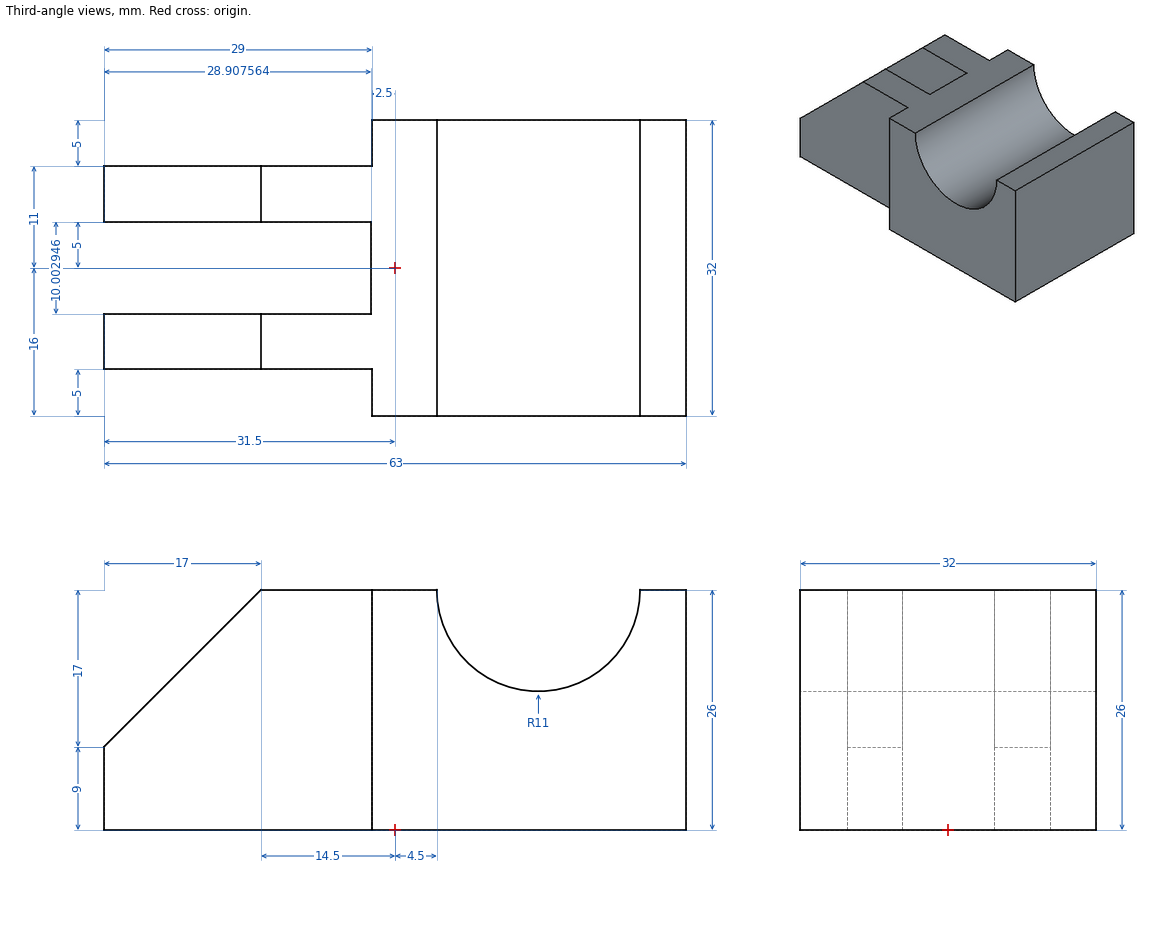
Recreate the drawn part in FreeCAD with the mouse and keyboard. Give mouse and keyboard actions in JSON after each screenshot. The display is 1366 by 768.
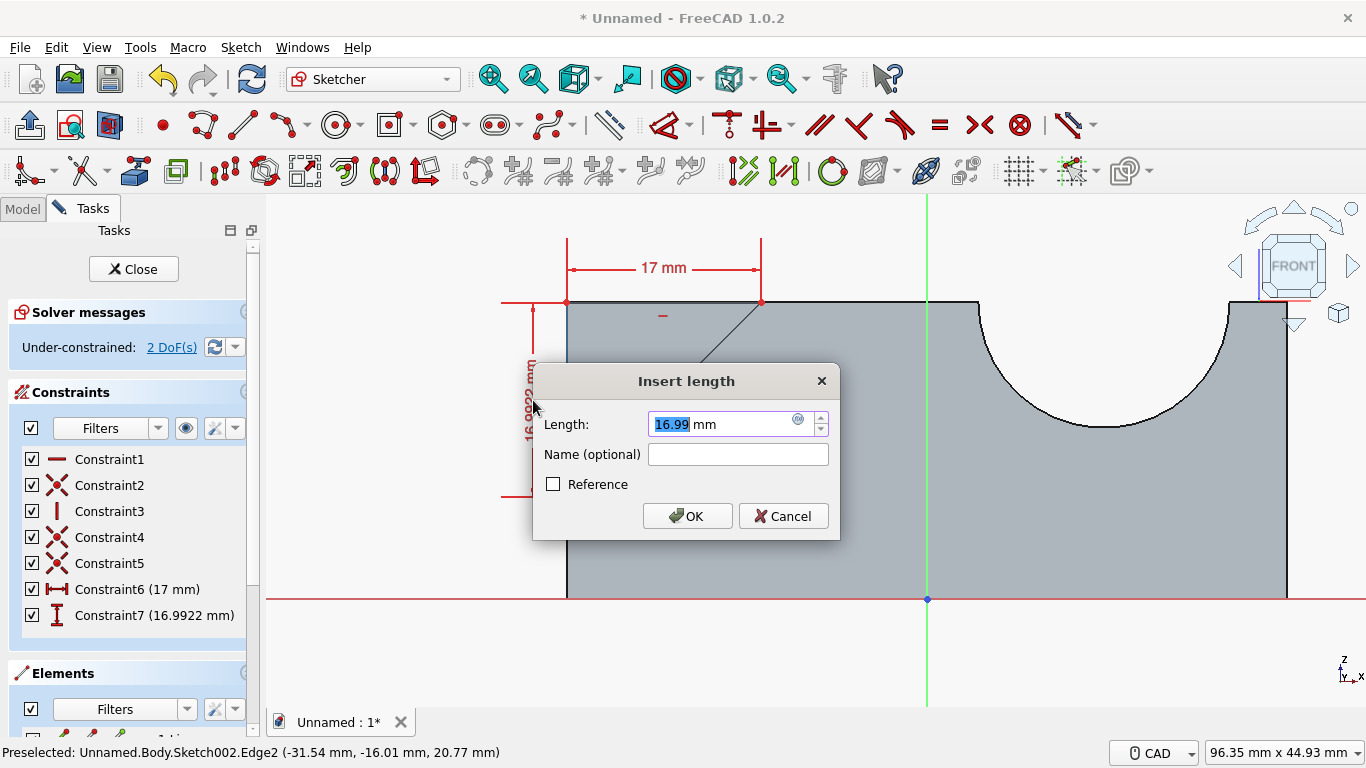
{"action": "type", "text": "17"}
{"action": "key", "text": "Return"}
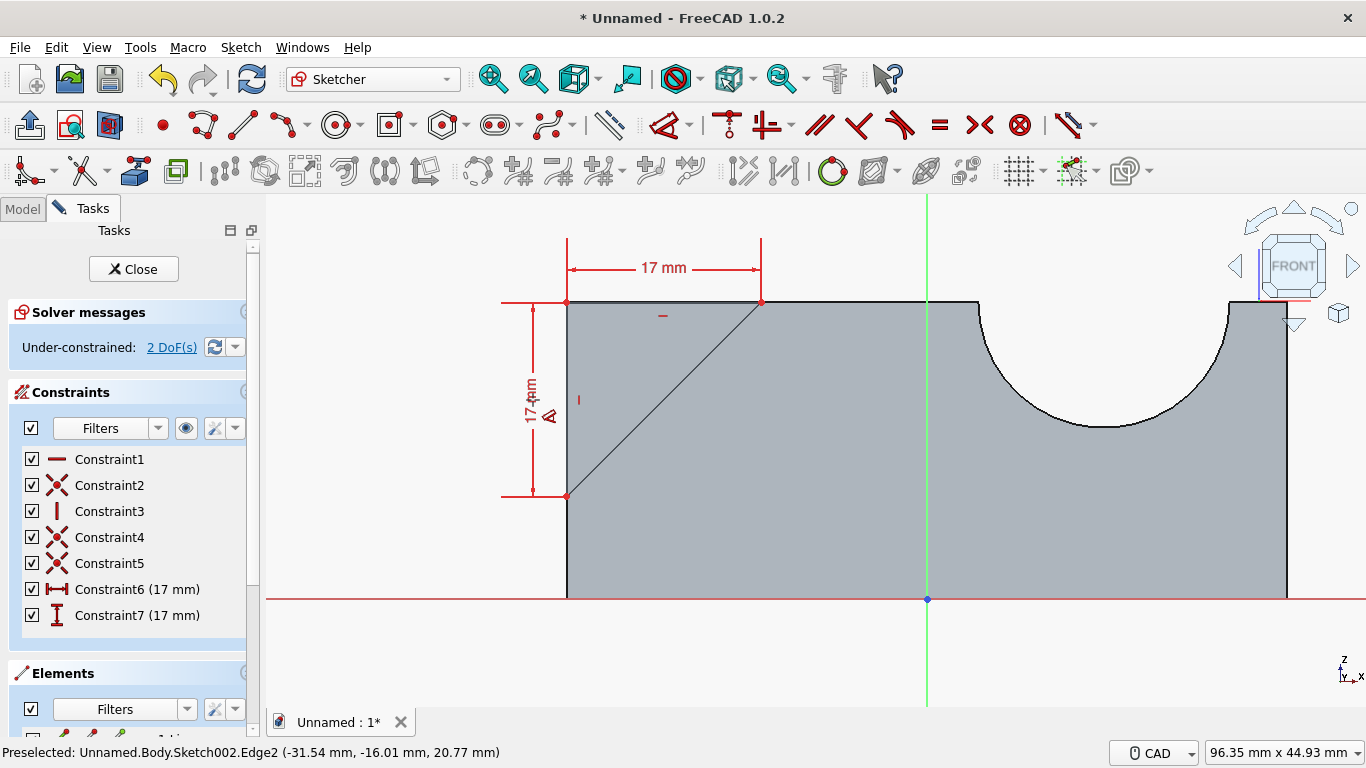
{"action": "left_click", "coordinate": [567, 497]}
{"action": "left_click", "coordinate": [533, 548]}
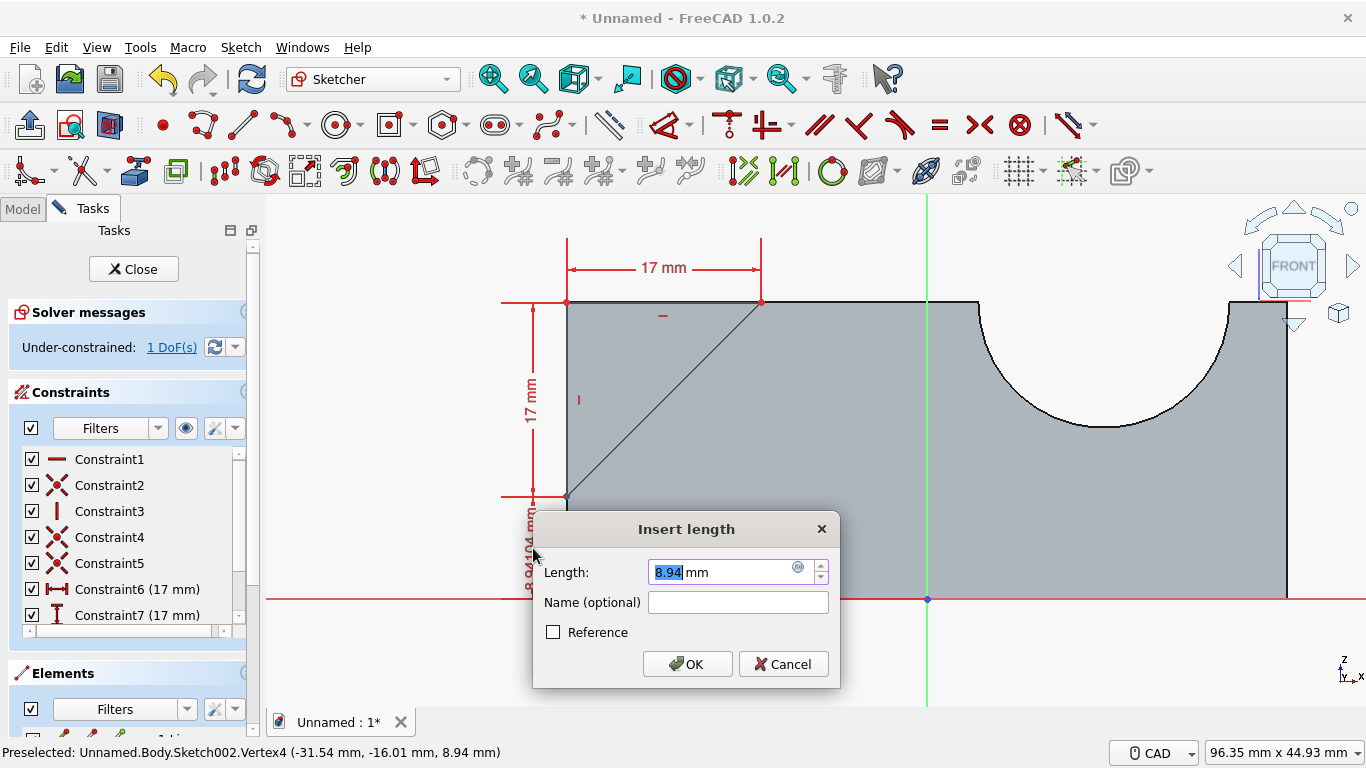
{"action": "type", "text": "9"}
{"action": "key", "text": "Return"}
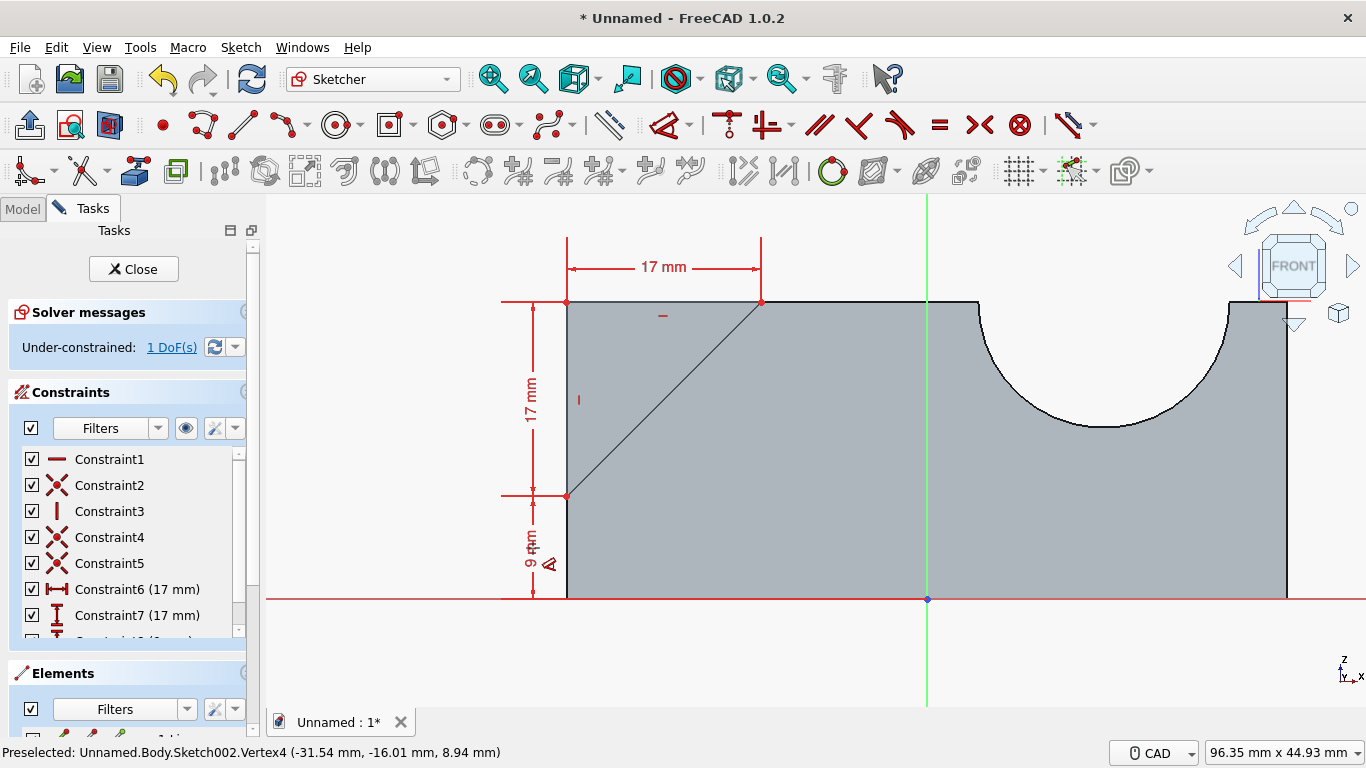
{"action": "left_click", "coordinate": [761, 302]}
{"action": "left_click", "coordinate": [844, 633]}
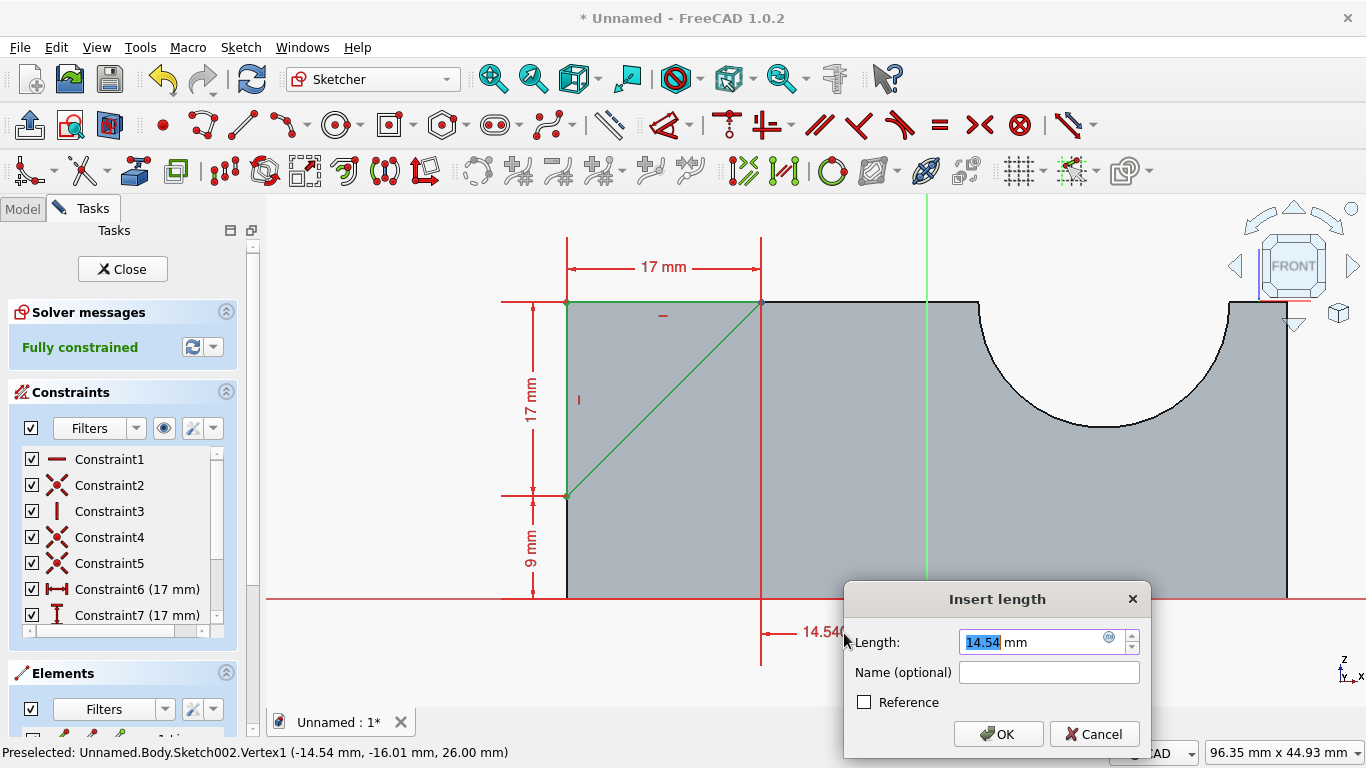
{"action": "type", "text": "14.5"}
{"action": "key", "text": "Return"}
{"action": "key", "text": "Escape"}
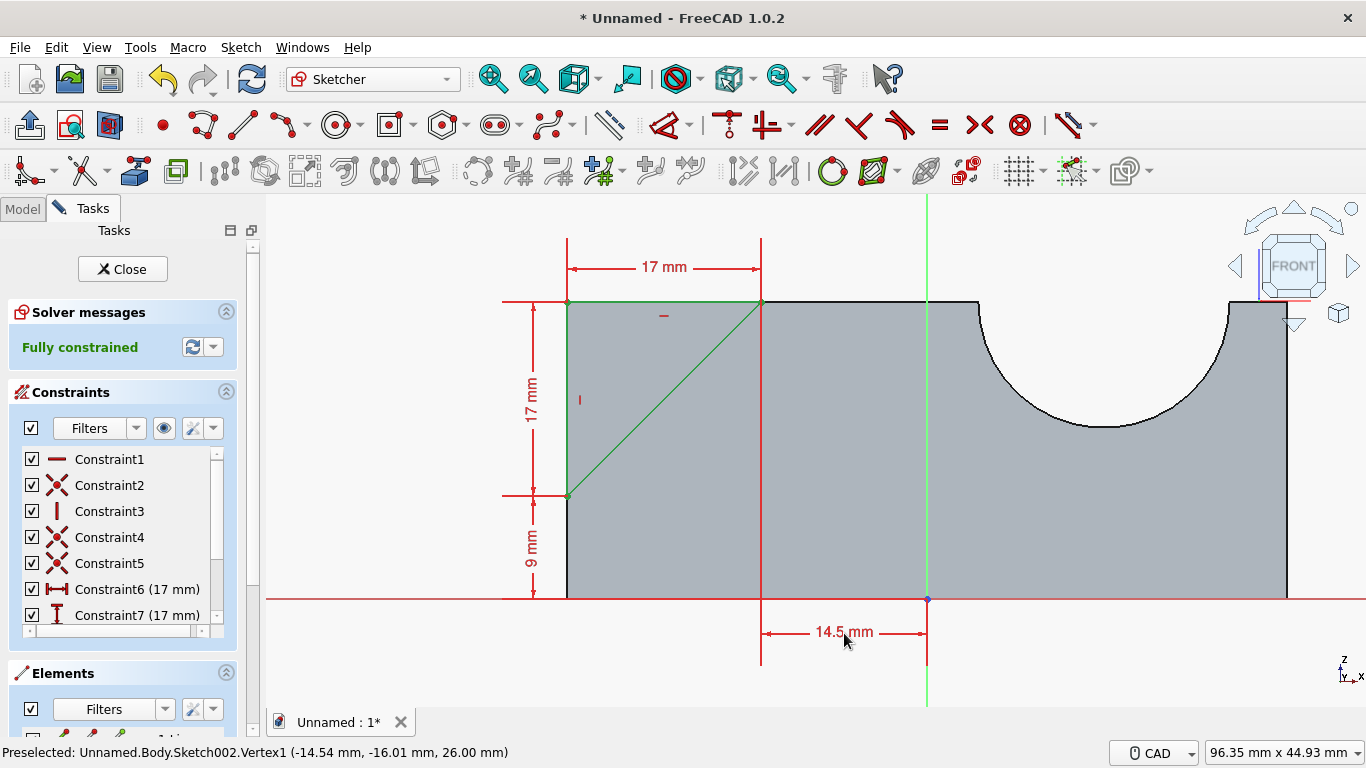
{"action": "left_click", "coordinate": [123, 269]}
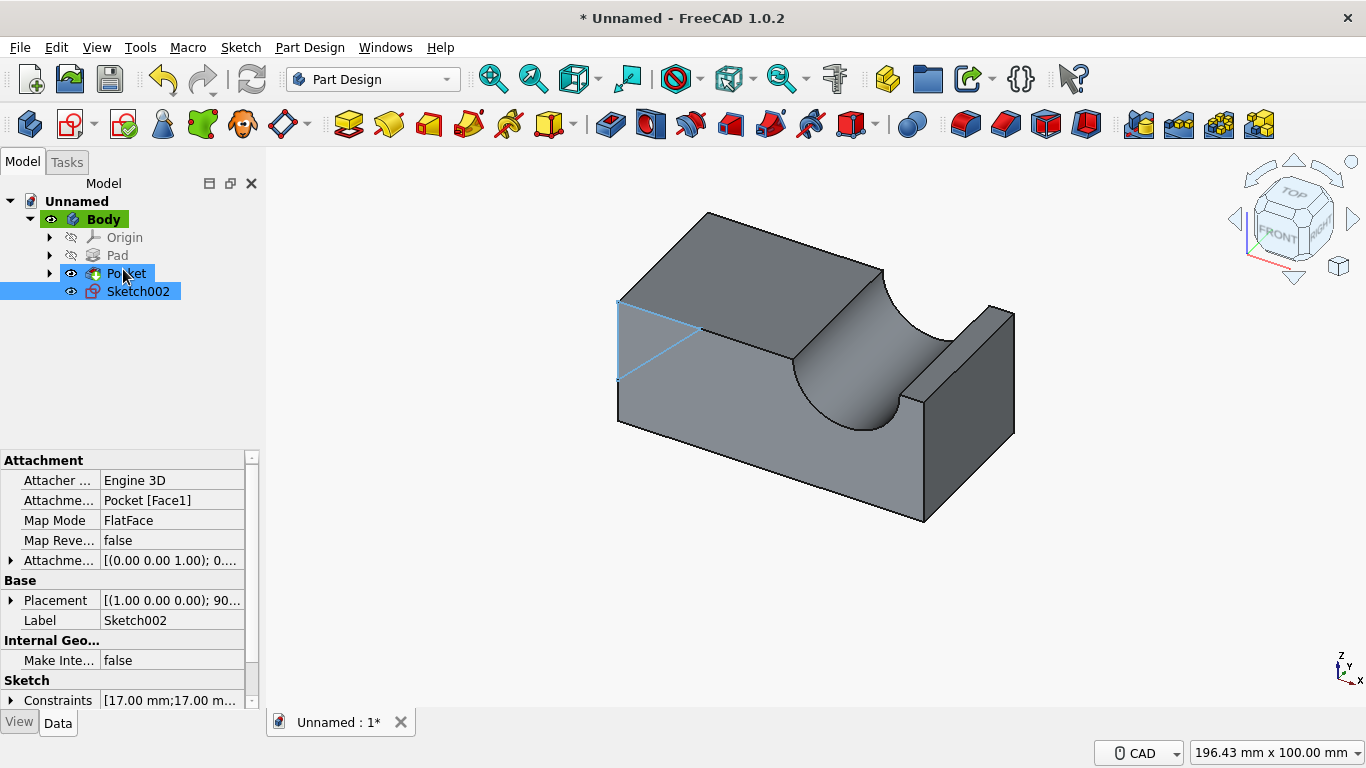
{"action": "left_click", "coordinate": [612, 124]}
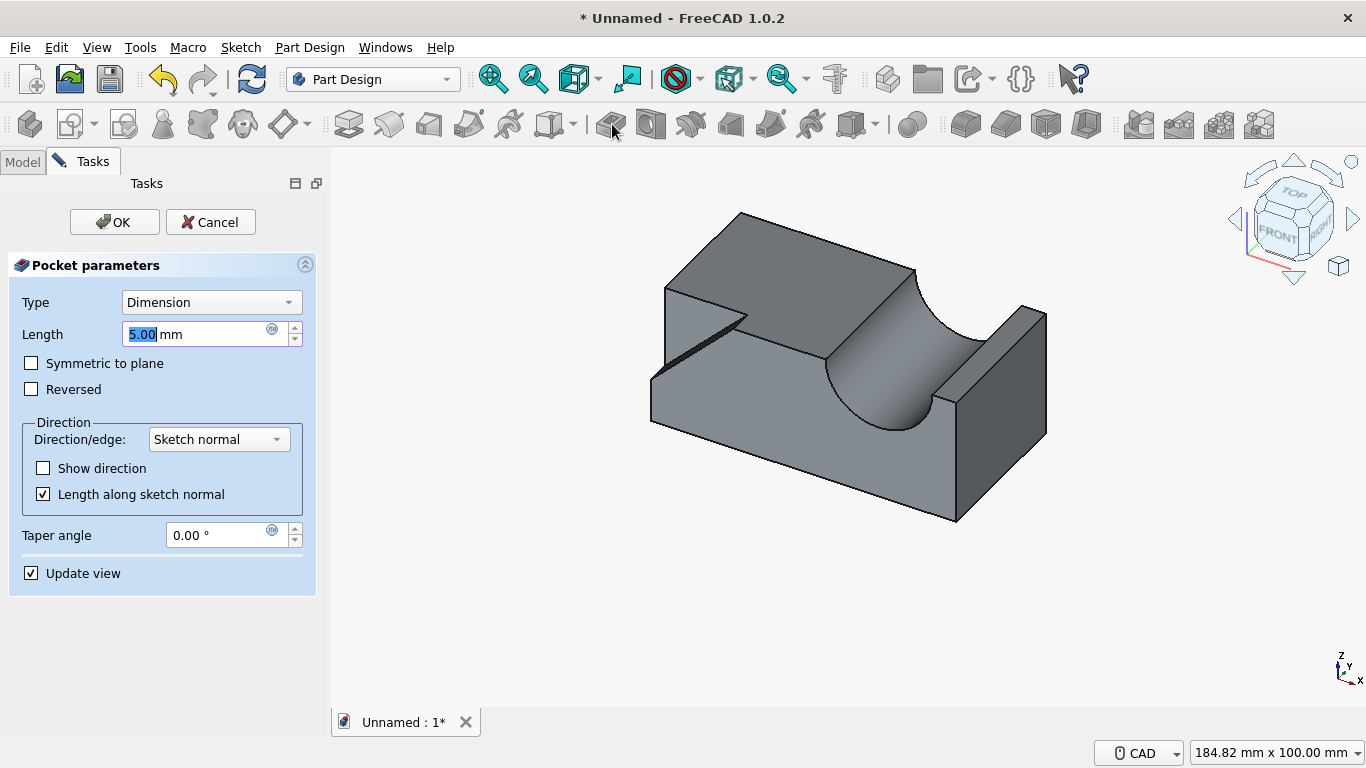
{"action": "type", "text": "32"}
{"action": "key", "text": "Tab"}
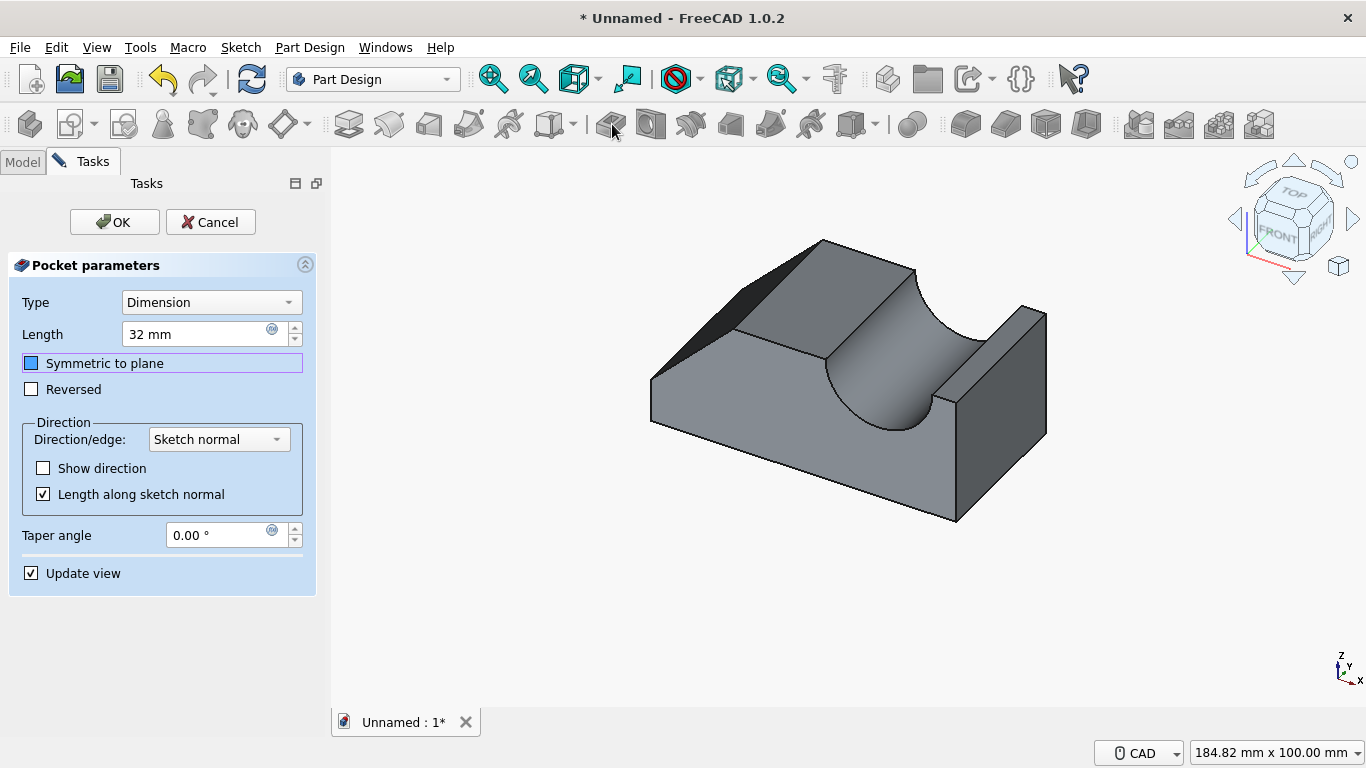
{"action": "left_click", "coordinate": [115, 222]}